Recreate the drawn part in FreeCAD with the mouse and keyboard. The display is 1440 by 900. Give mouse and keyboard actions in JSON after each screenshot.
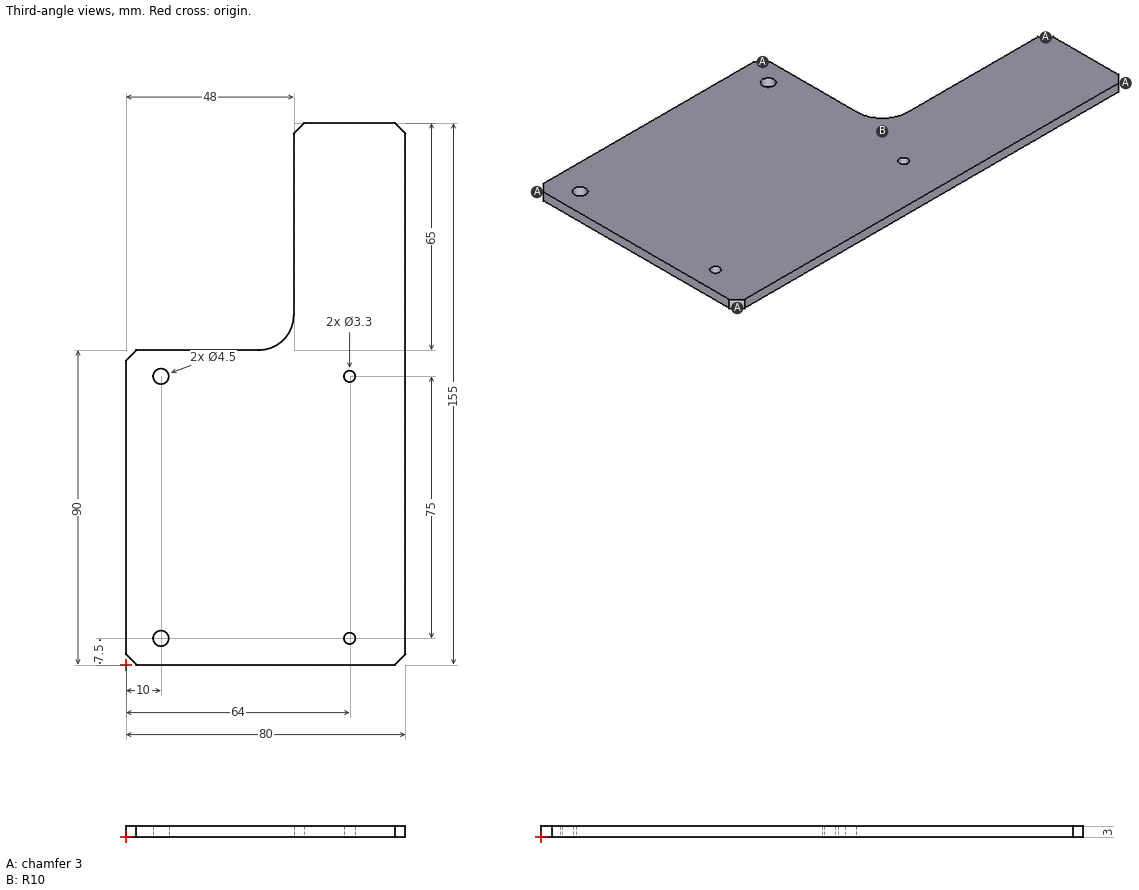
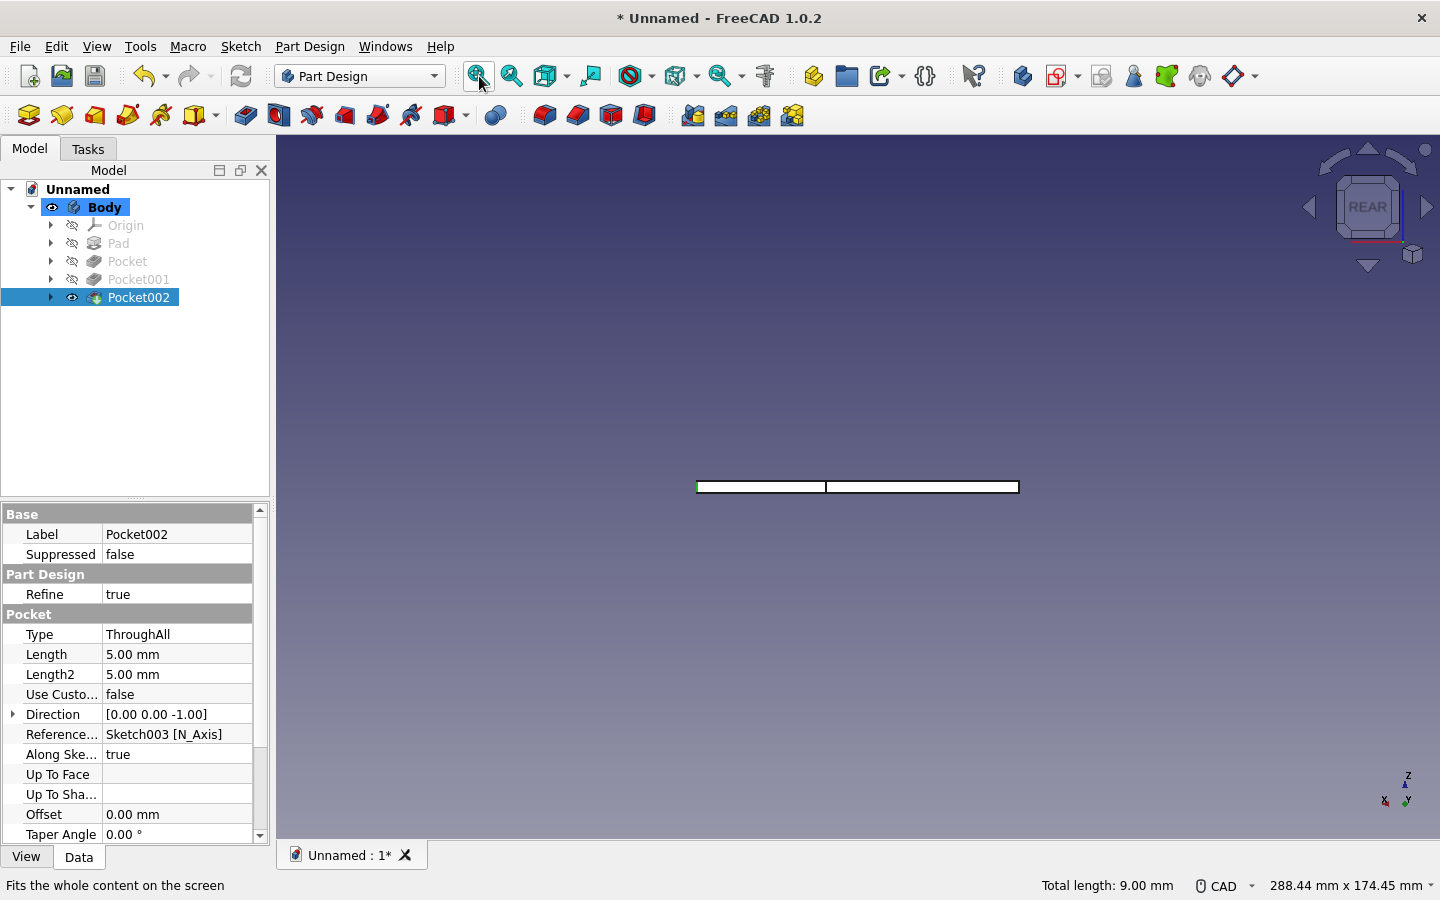
{"action": "left_click", "coordinate": [826, 486], "text": "ctrl"}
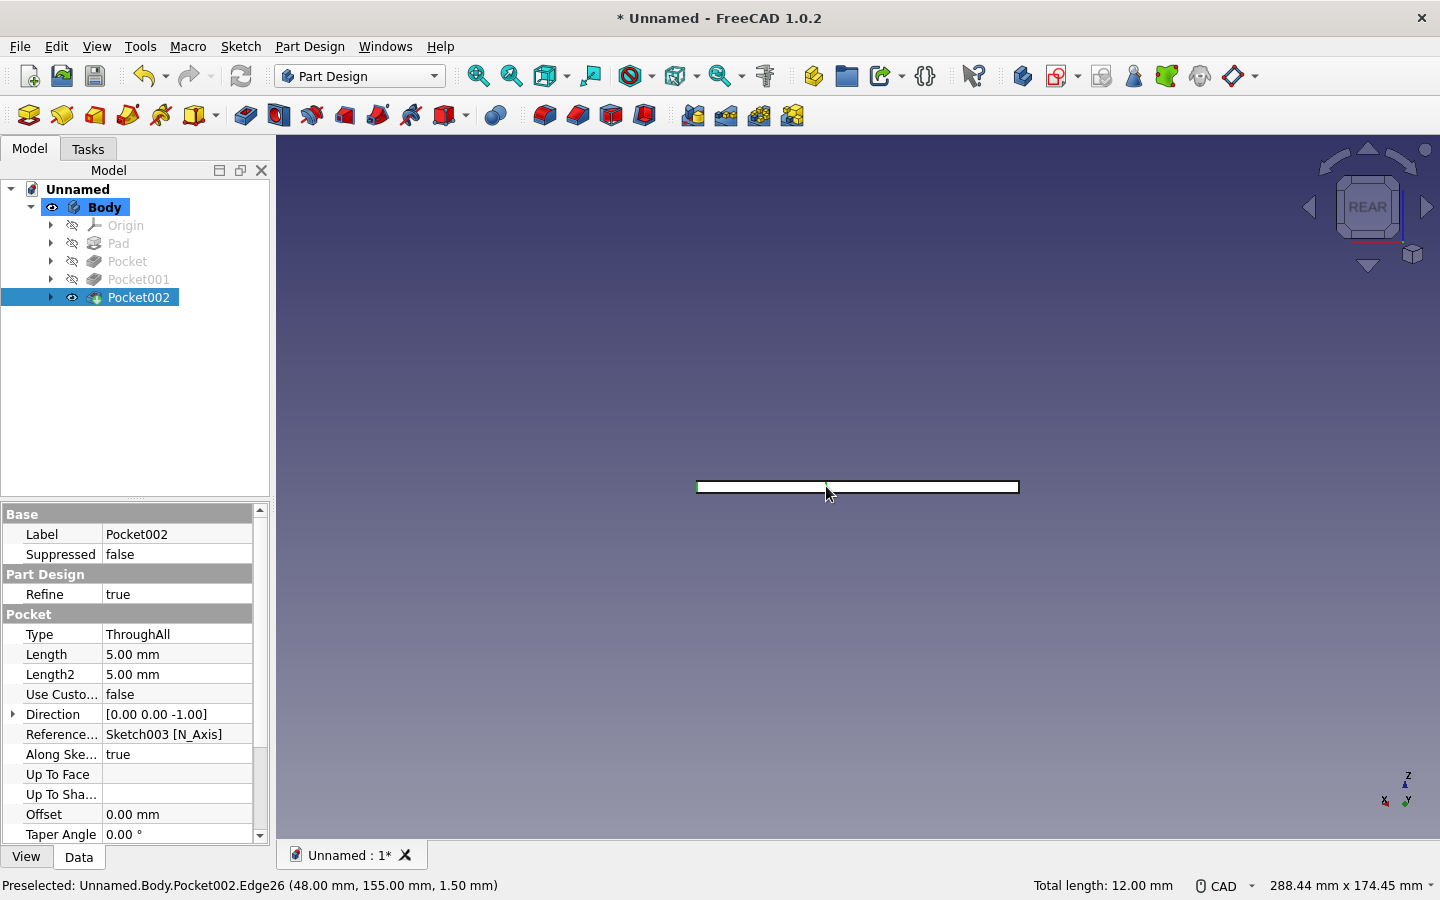
{"action": "left_click", "coordinate": [1019, 486], "text": "ctrl"}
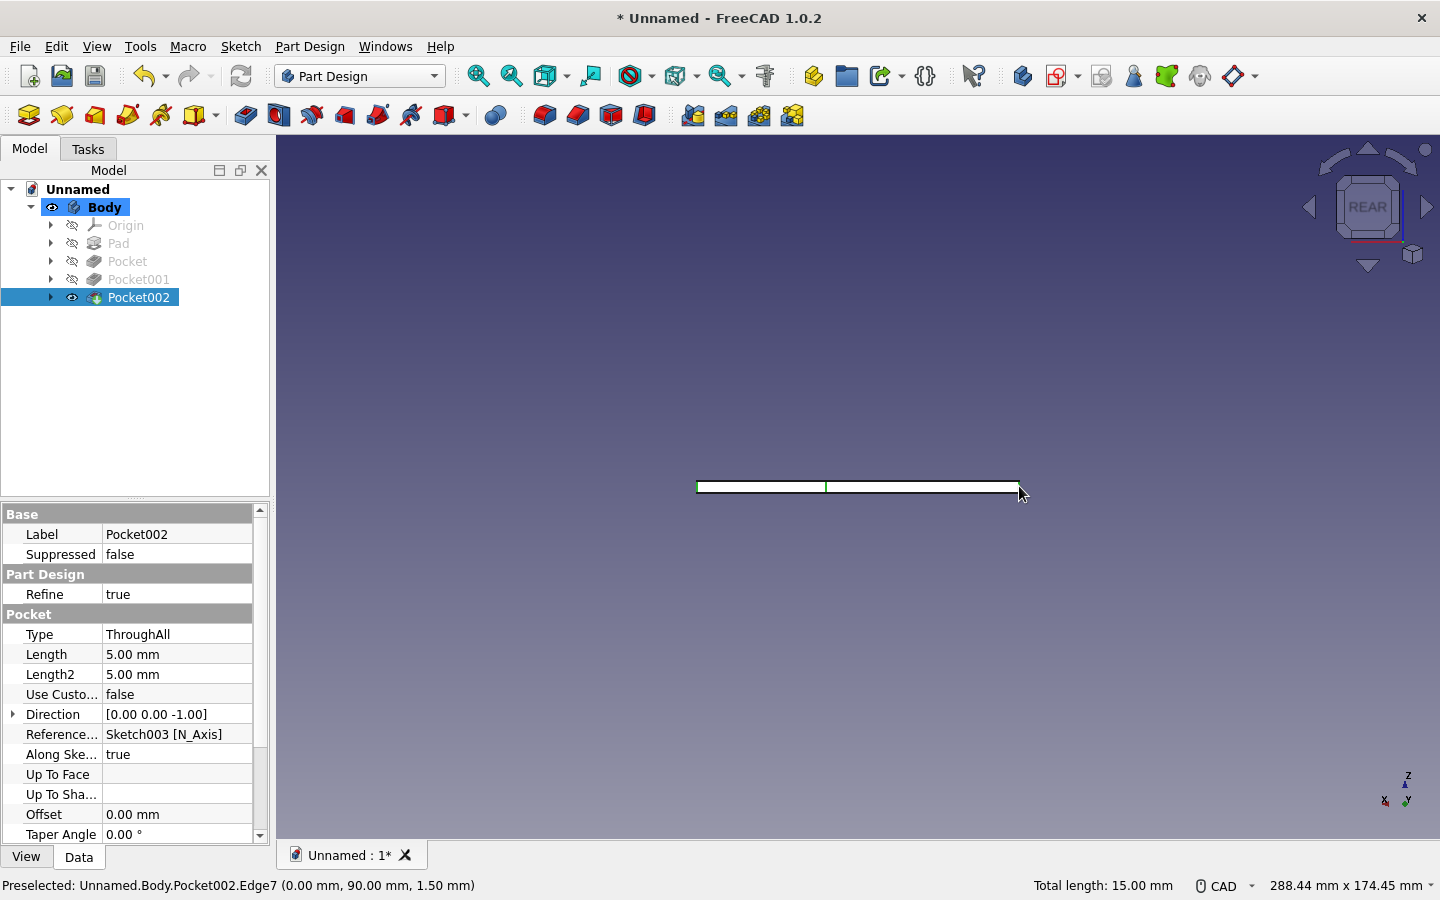
{"action": "left_click", "coordinate": [578, 116]}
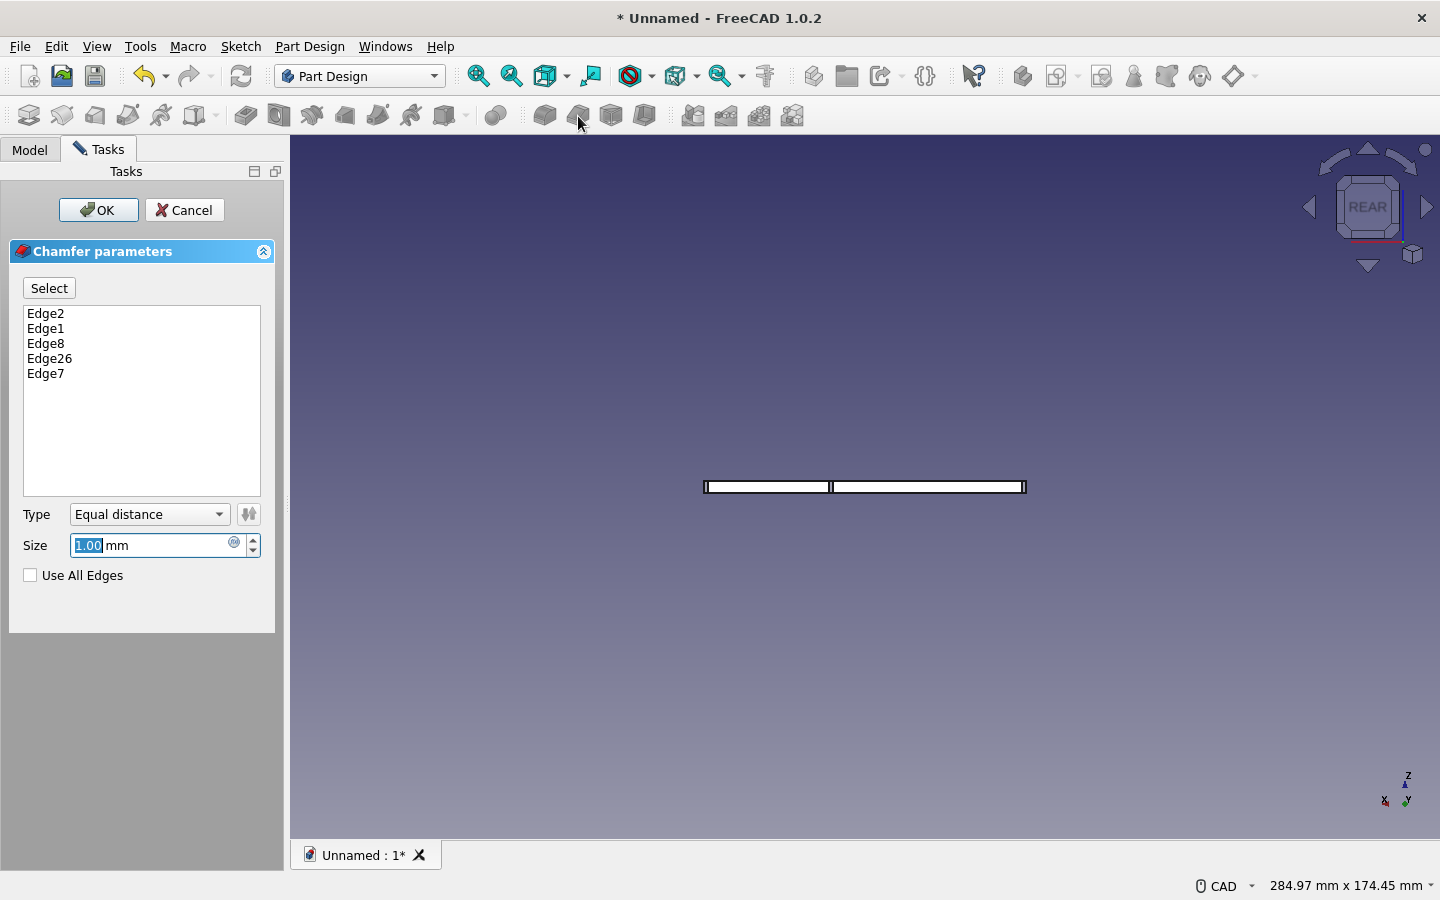
{"action": "type", "text": "3"}
{"action": "key", "text": "Tab"}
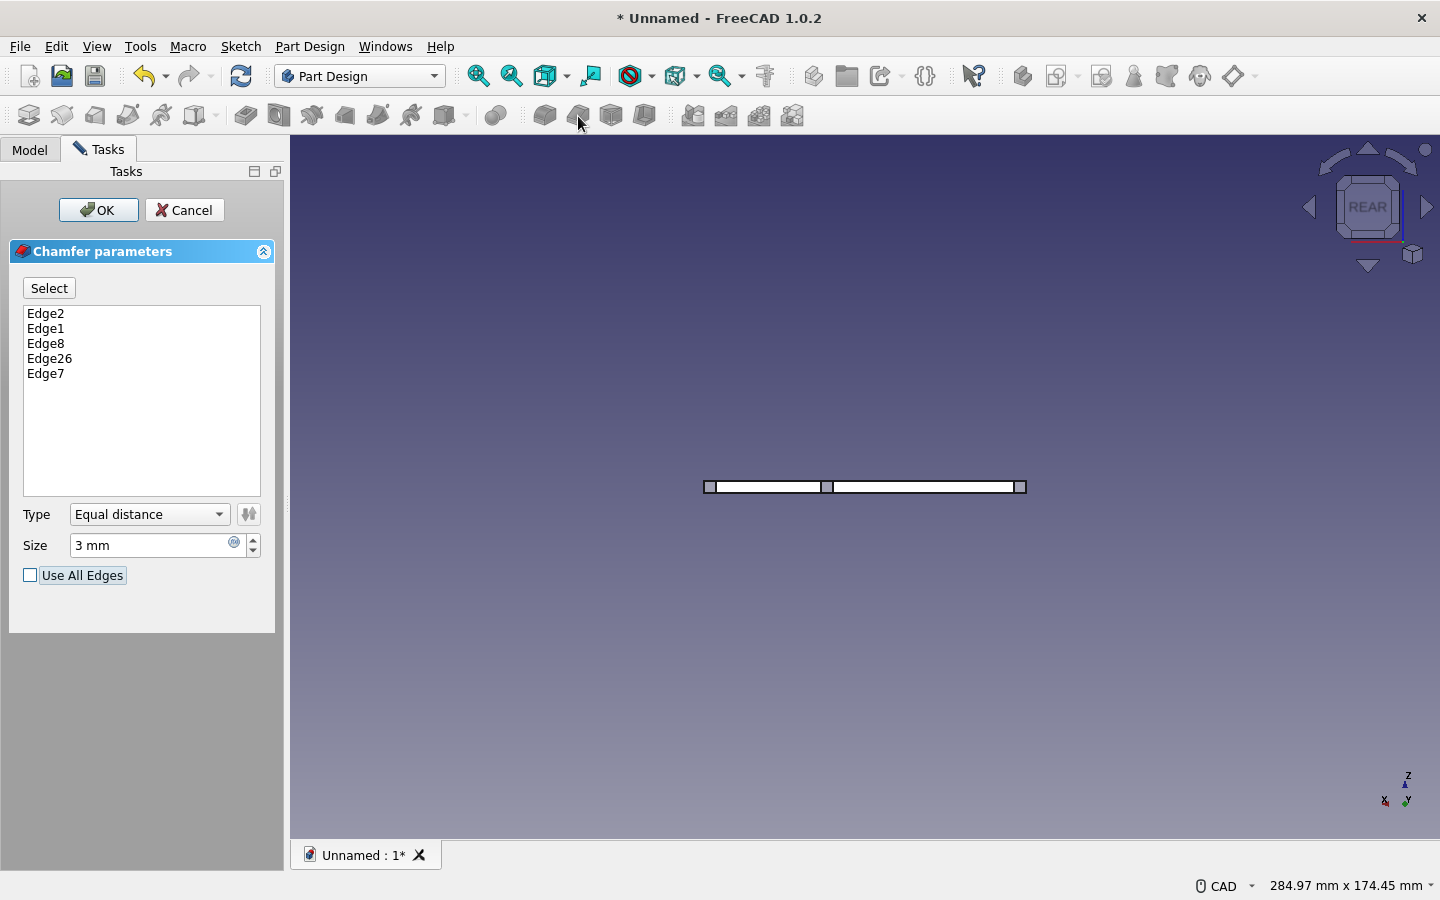
{"action": "left_click", "coordinate": [99, 210]}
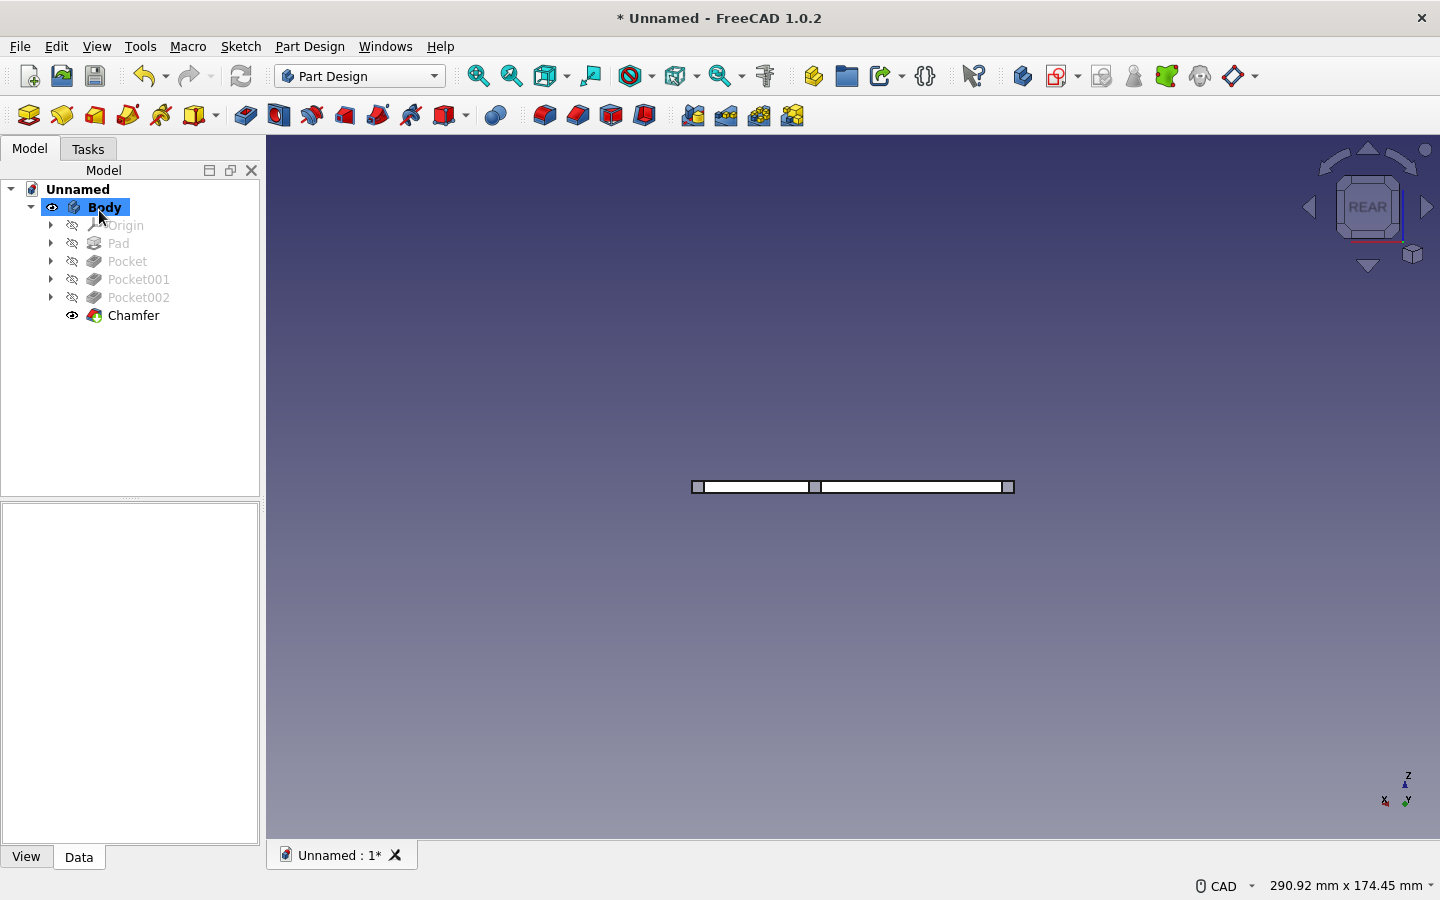
{"action": "left_click", "coordinate": [479, 76]}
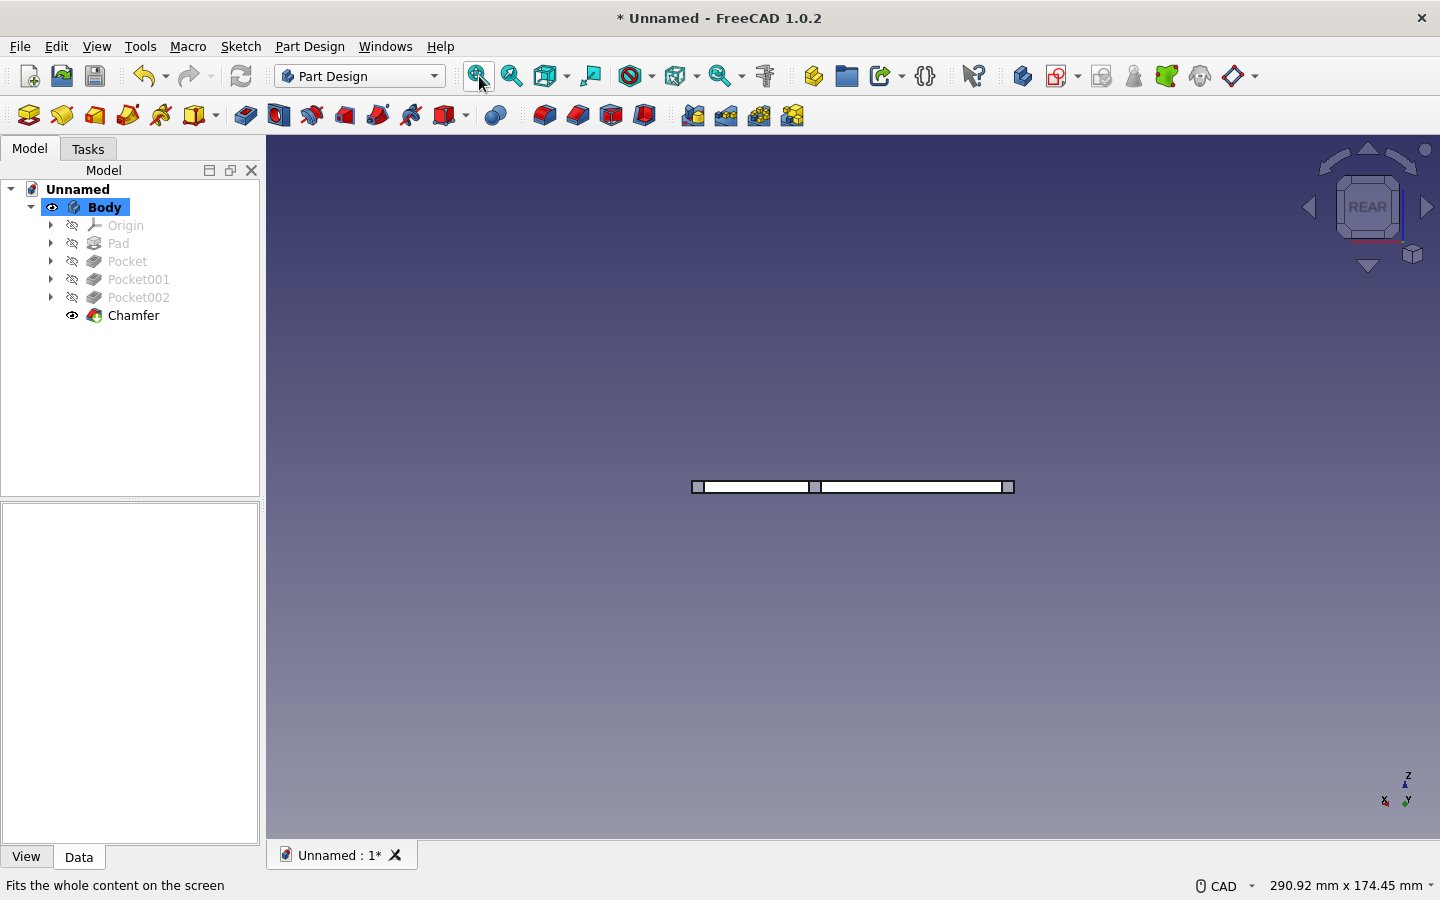
{"action": "scroll", "coordinate": [821, 486], "scroll_direction": "up", "scroll_amount": 6}